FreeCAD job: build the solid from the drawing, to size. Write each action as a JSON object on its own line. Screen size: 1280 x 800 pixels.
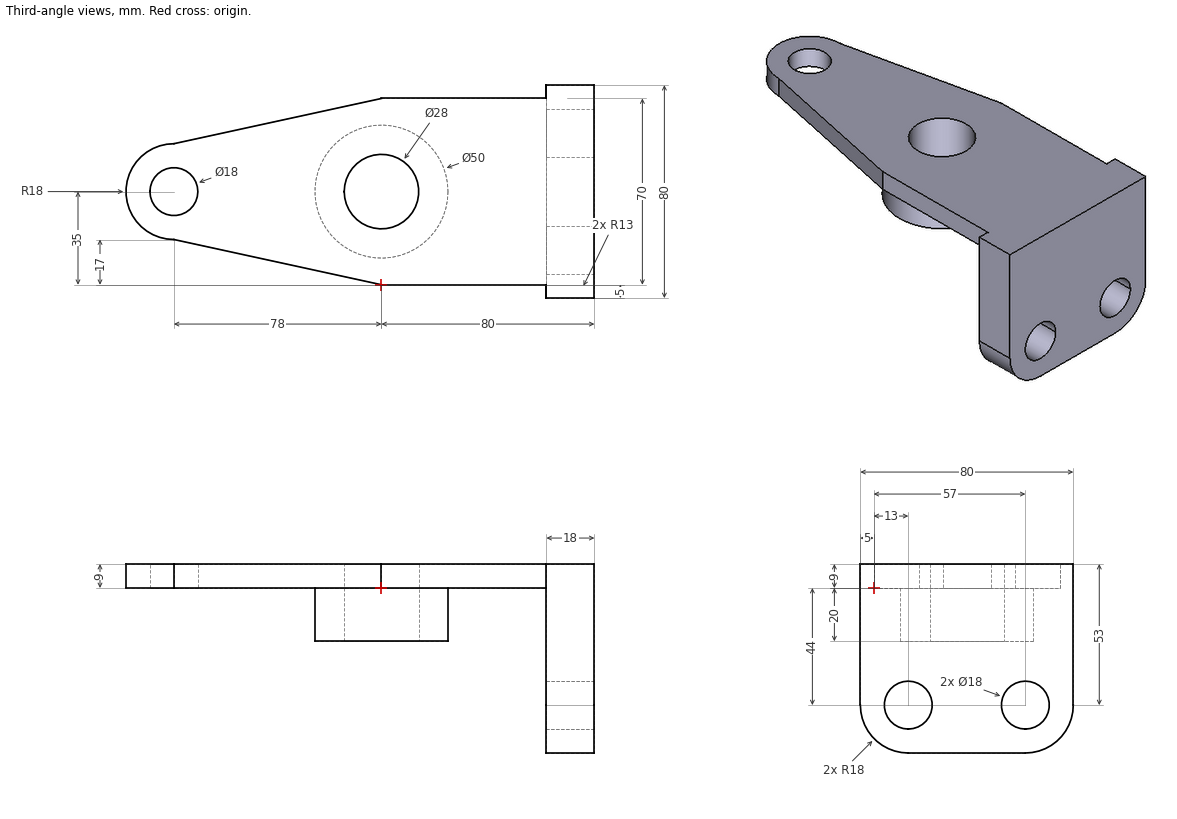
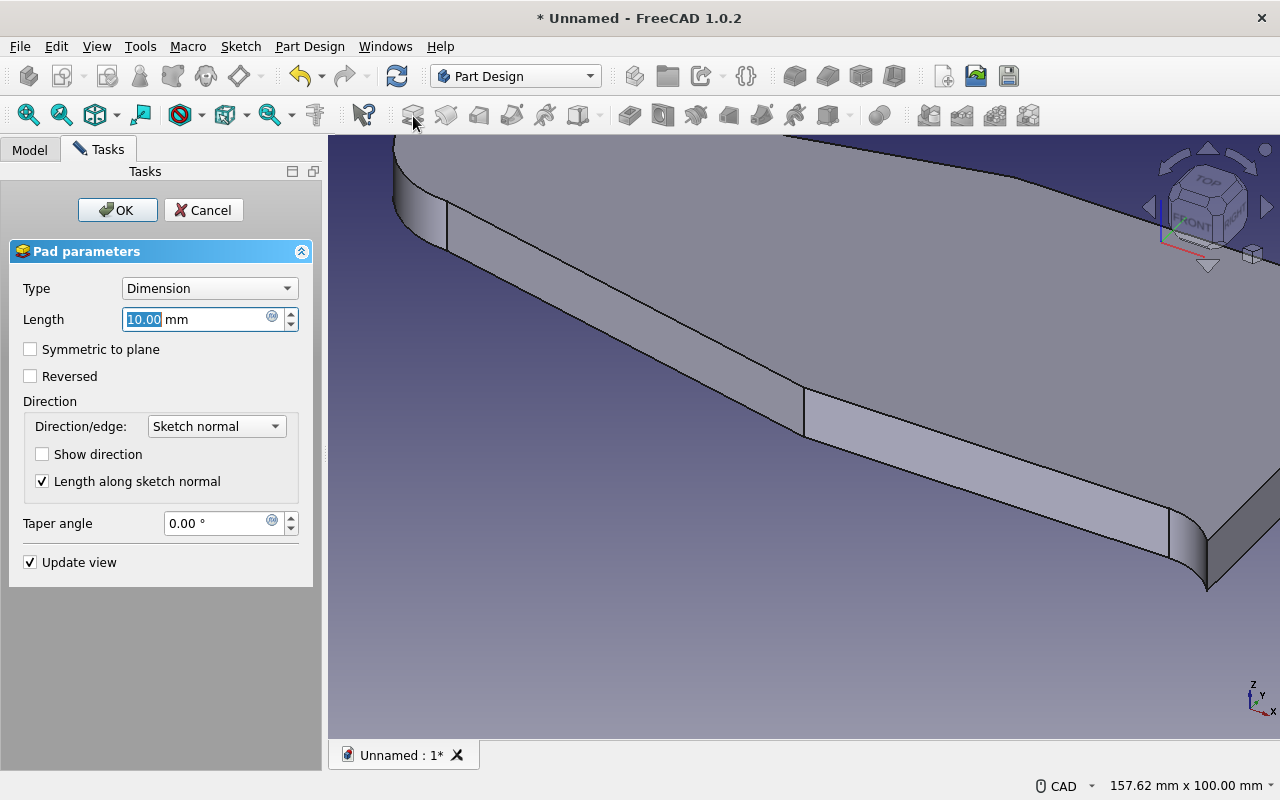
{"action": "type", "text": "9"}
{"action": "key", "text": "Tab"}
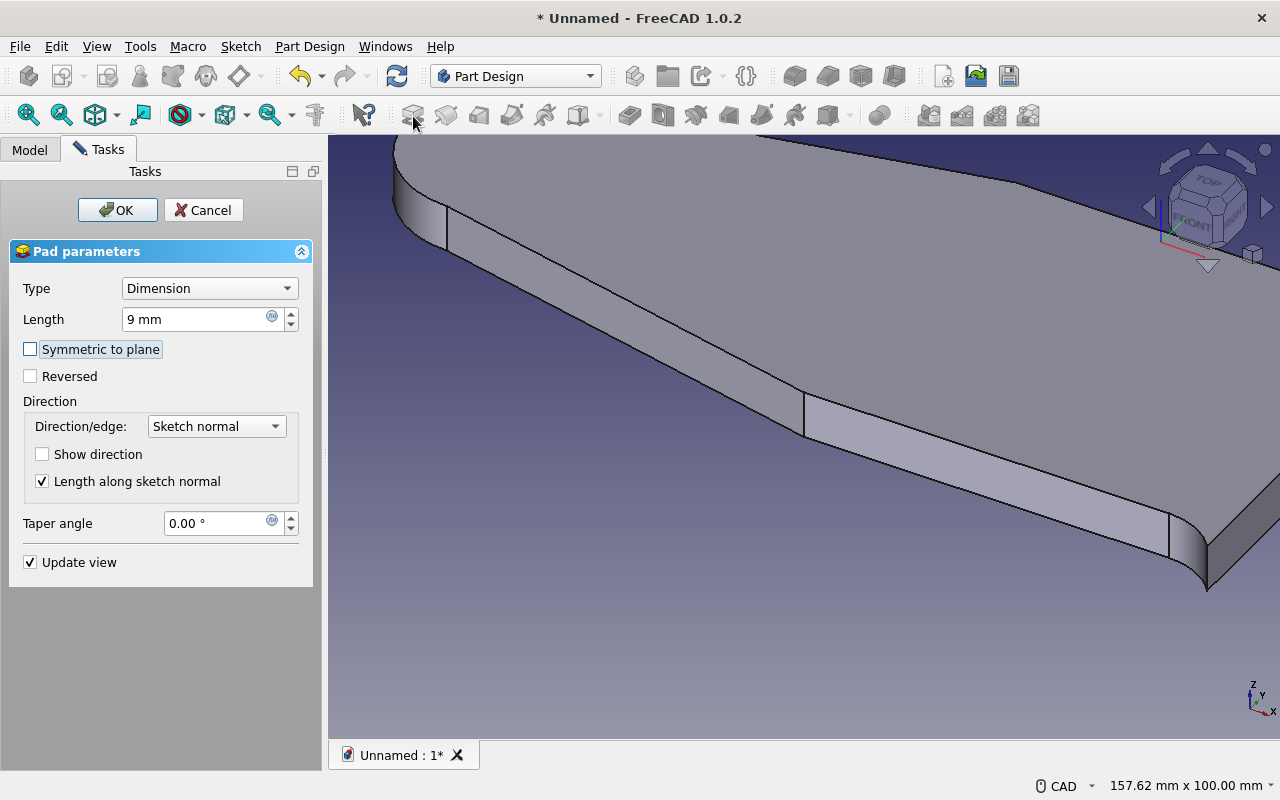
{"action": "left_click", "coordinate": [118, 210]}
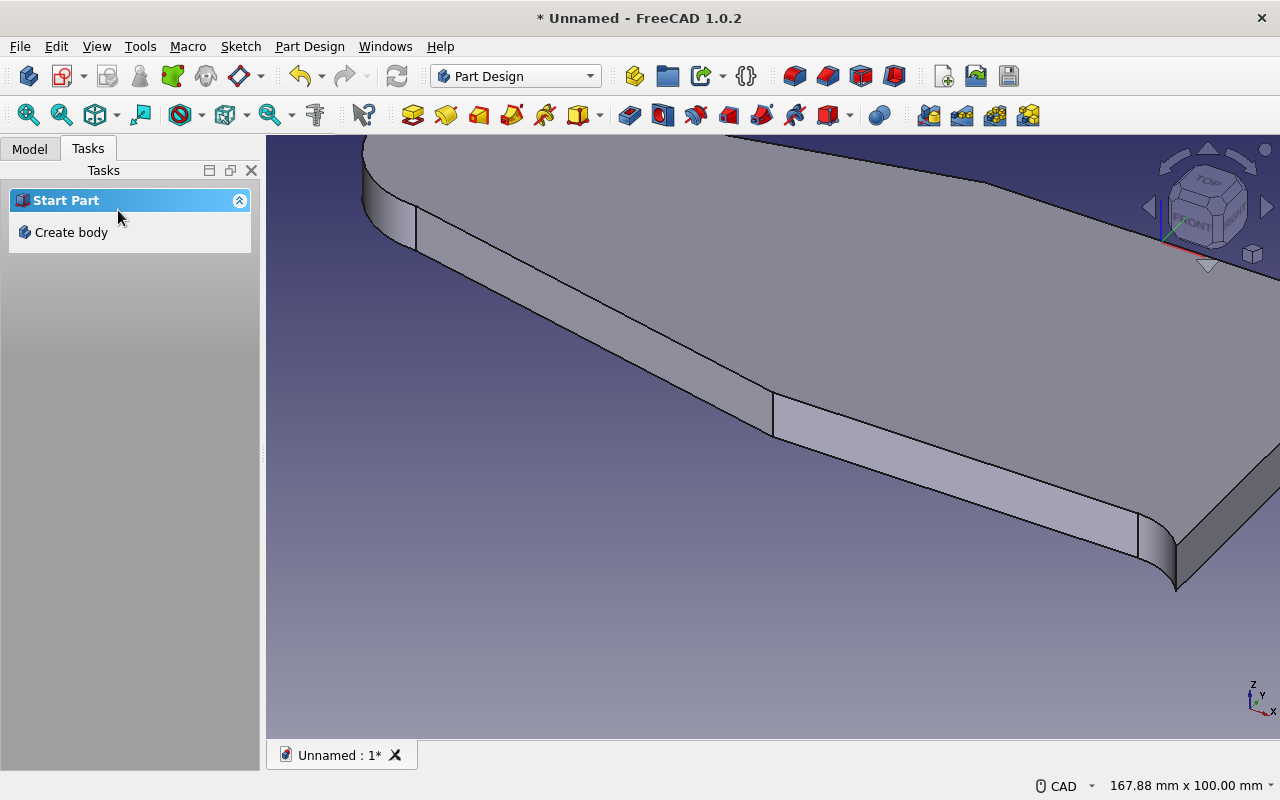
{"action": "left_click", "coordinate": [29, 116]}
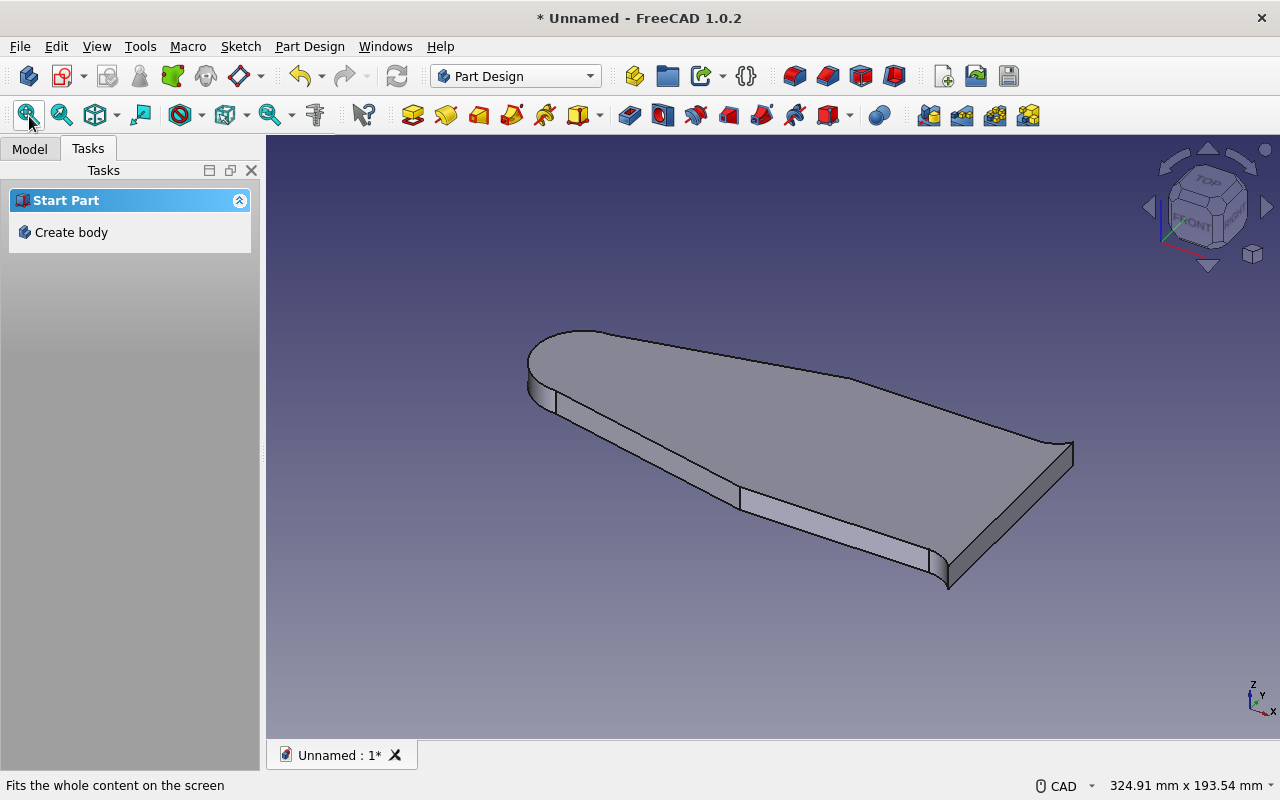
{"action": "key", "text": "5"}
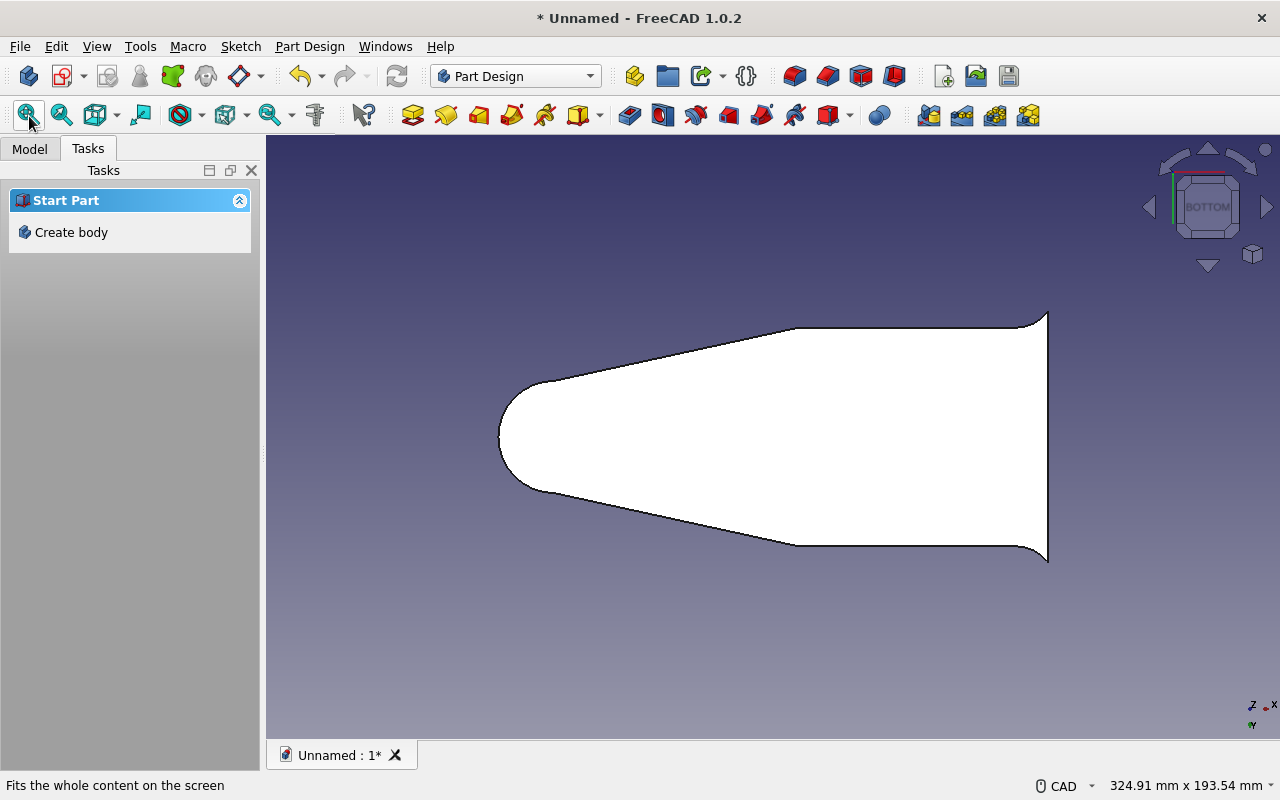
{"action": "left_click", "coordinate": [930, 436]}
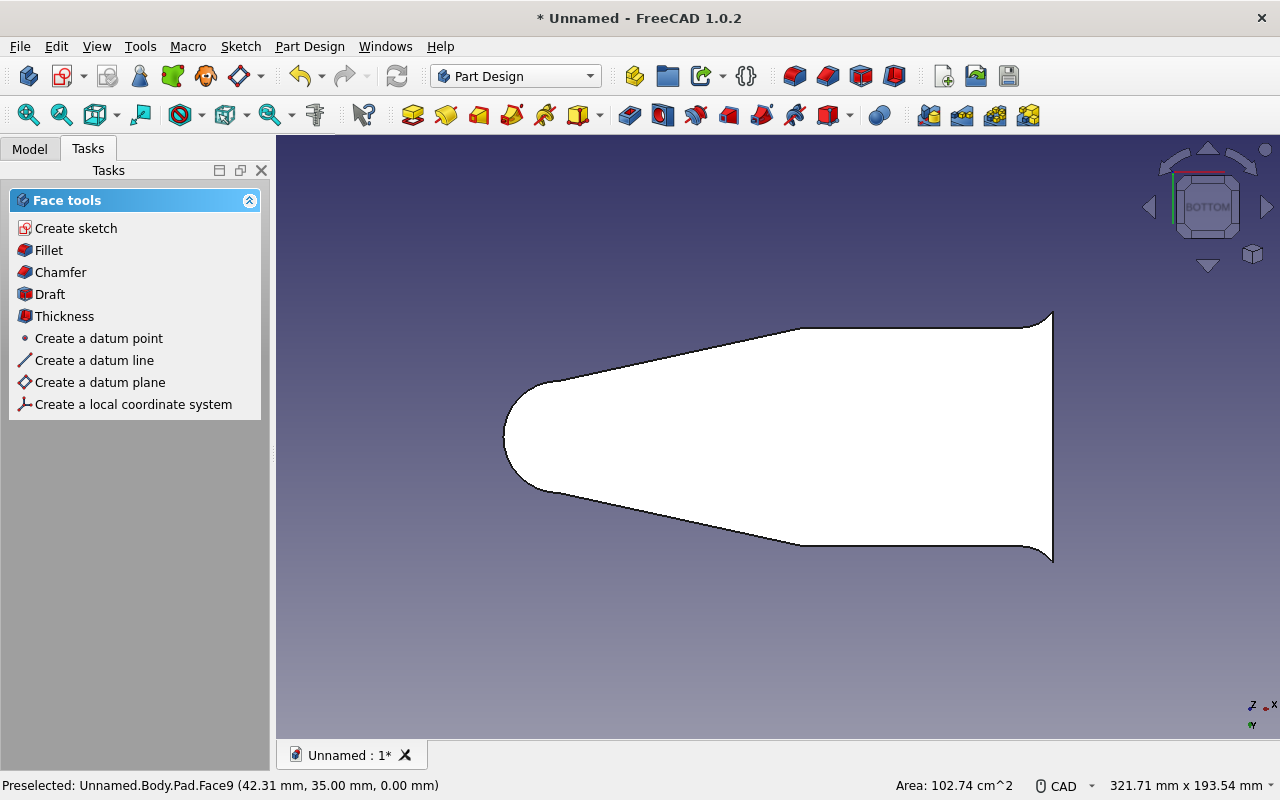
{"action": "left_click", "coordinate": [62, 76]}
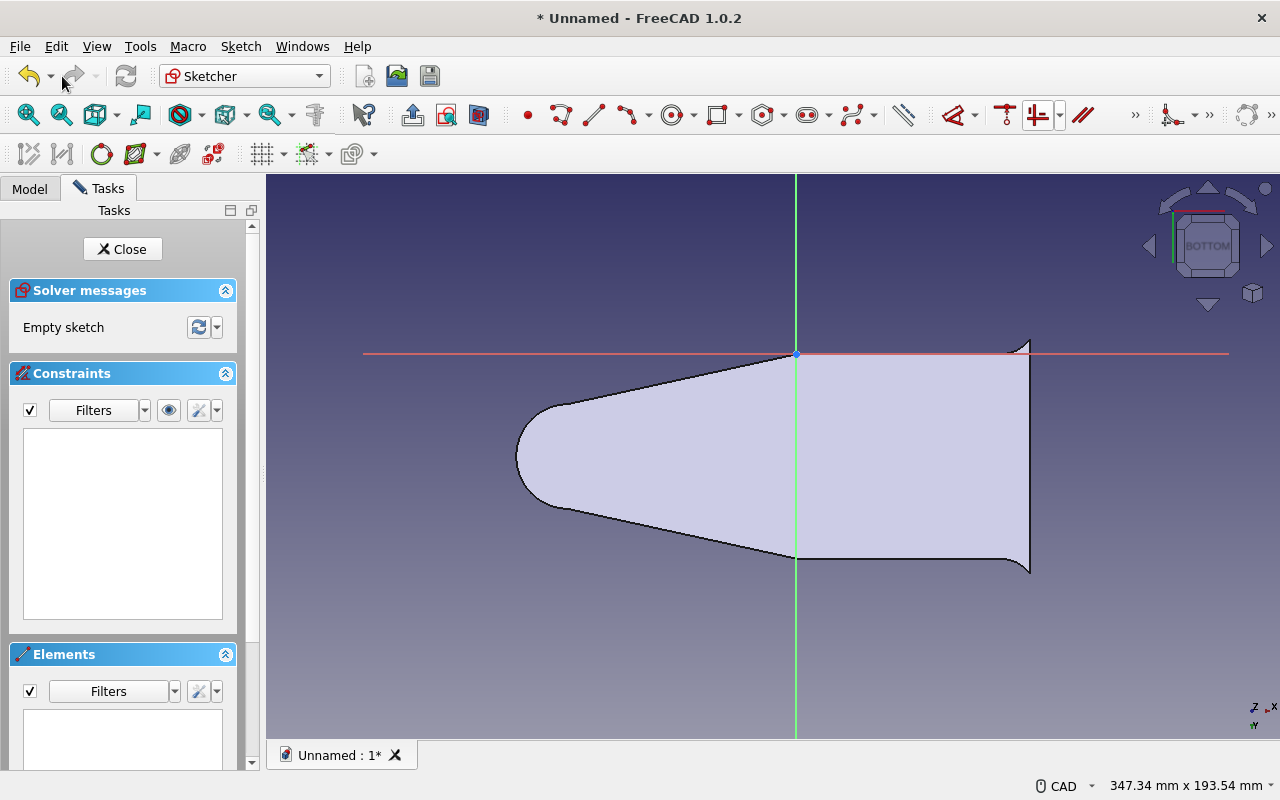
{"action": "scroll", "coordinate": [547, 456], "scroll_direction": "up", "scroll_amount": 10}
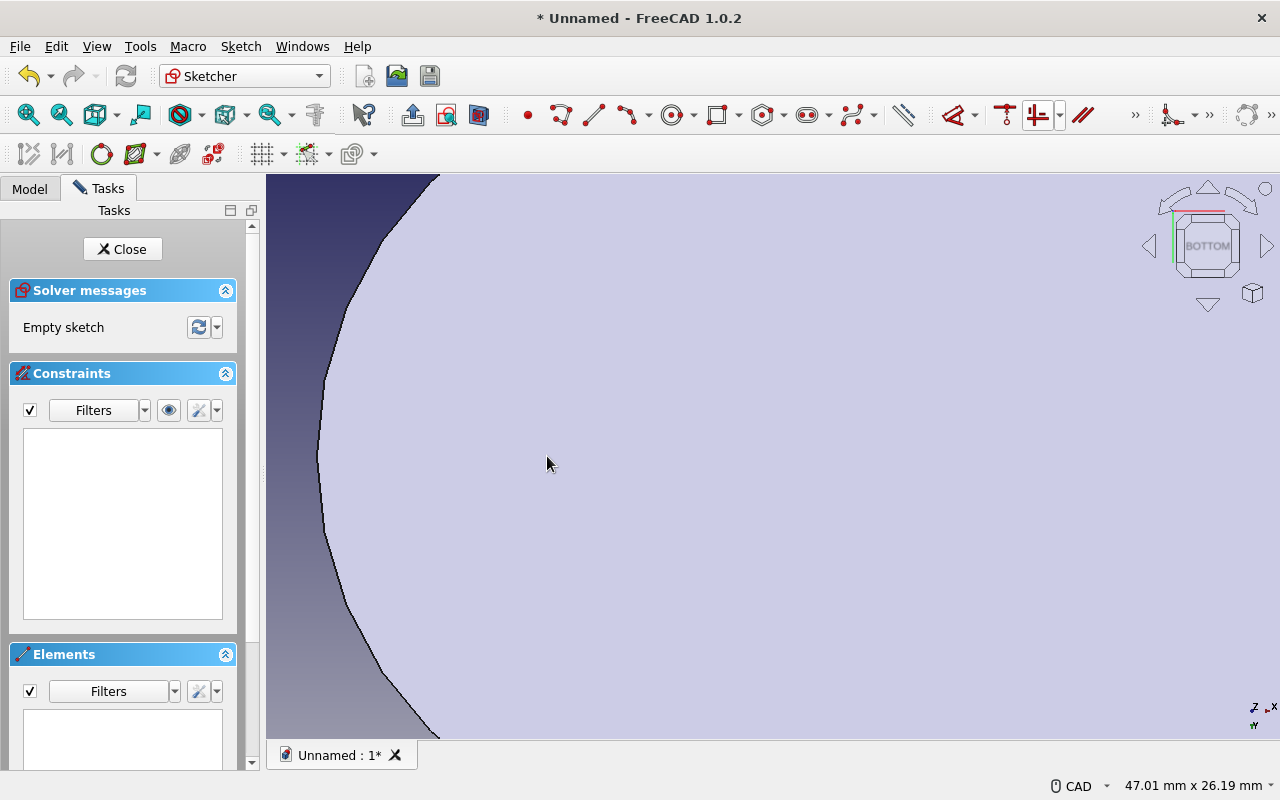
{"action": "key", "text": "g c"}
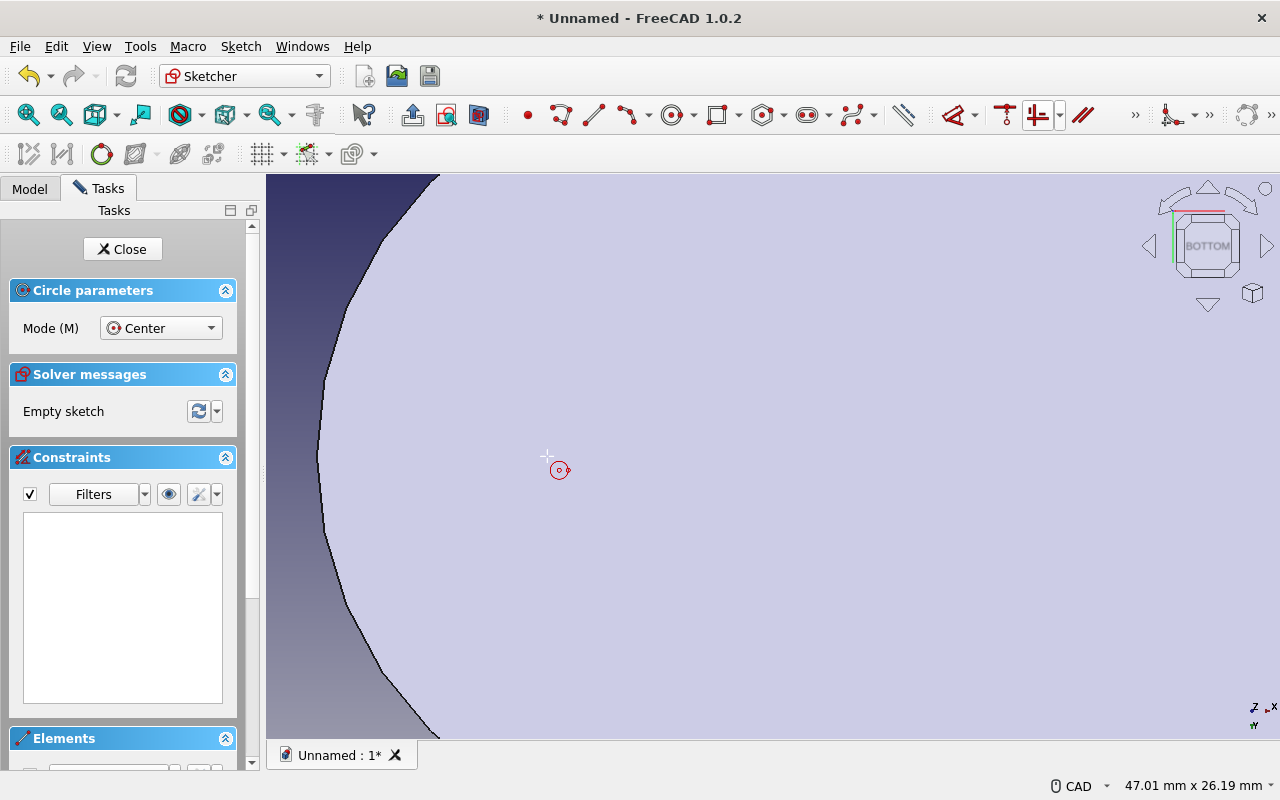
{"action": "left_click", "coordinate": [705, 456]}
{"action": "left_click", "coordinate": [842, 319]}
{"action": "key", "text": "Escape"}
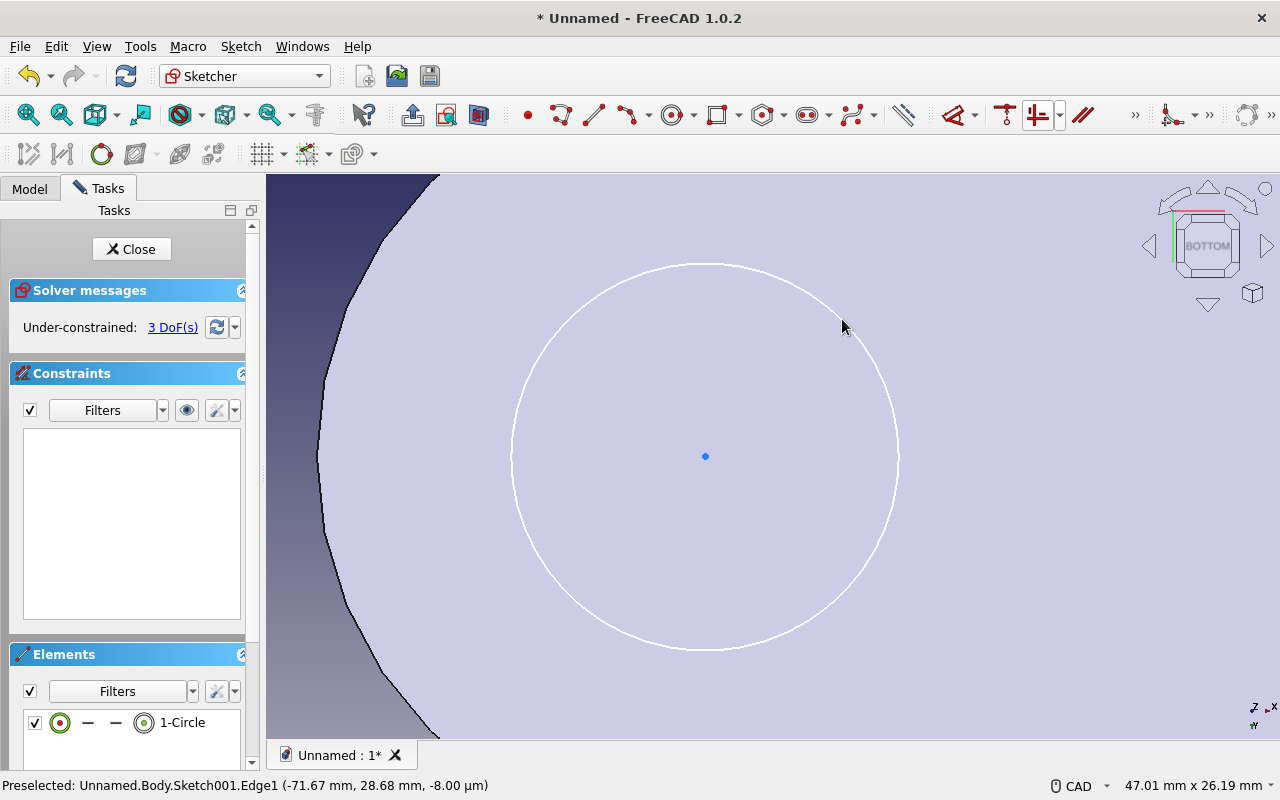
{"action": "left_click", "coordinate": [952, 116]}